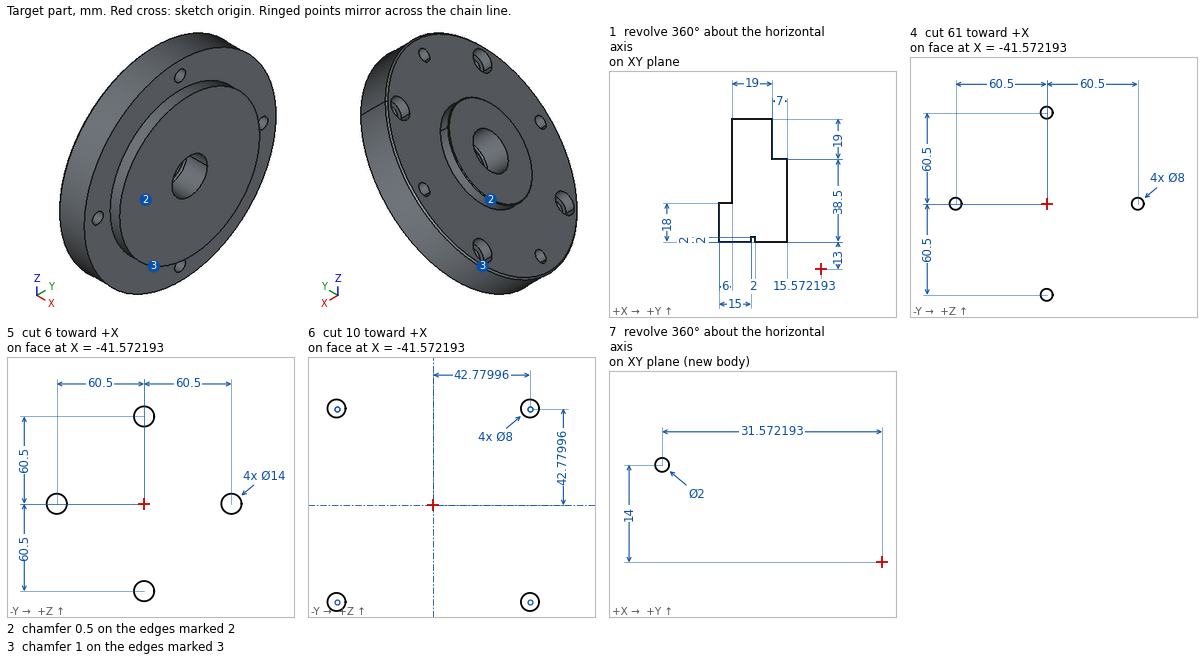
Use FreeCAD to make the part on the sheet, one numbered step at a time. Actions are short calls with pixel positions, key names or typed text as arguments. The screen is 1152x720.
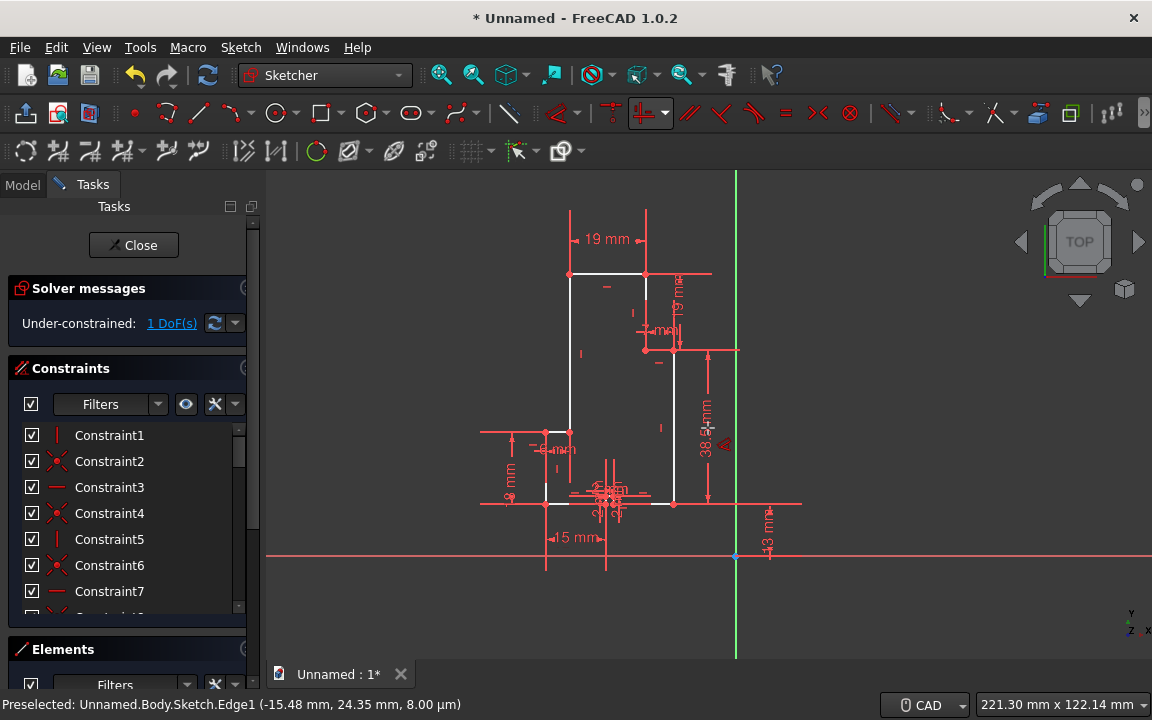
click(674, 504)
click(705, 590)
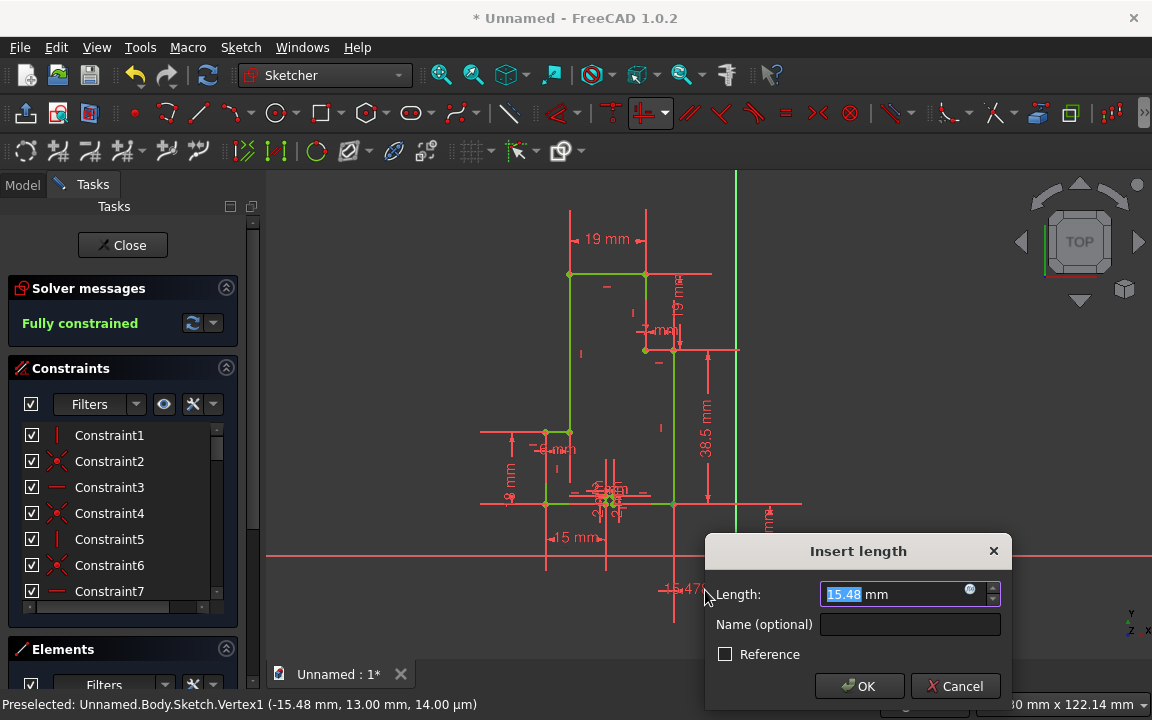
text(15.572193)
key(Return)
key(Escape)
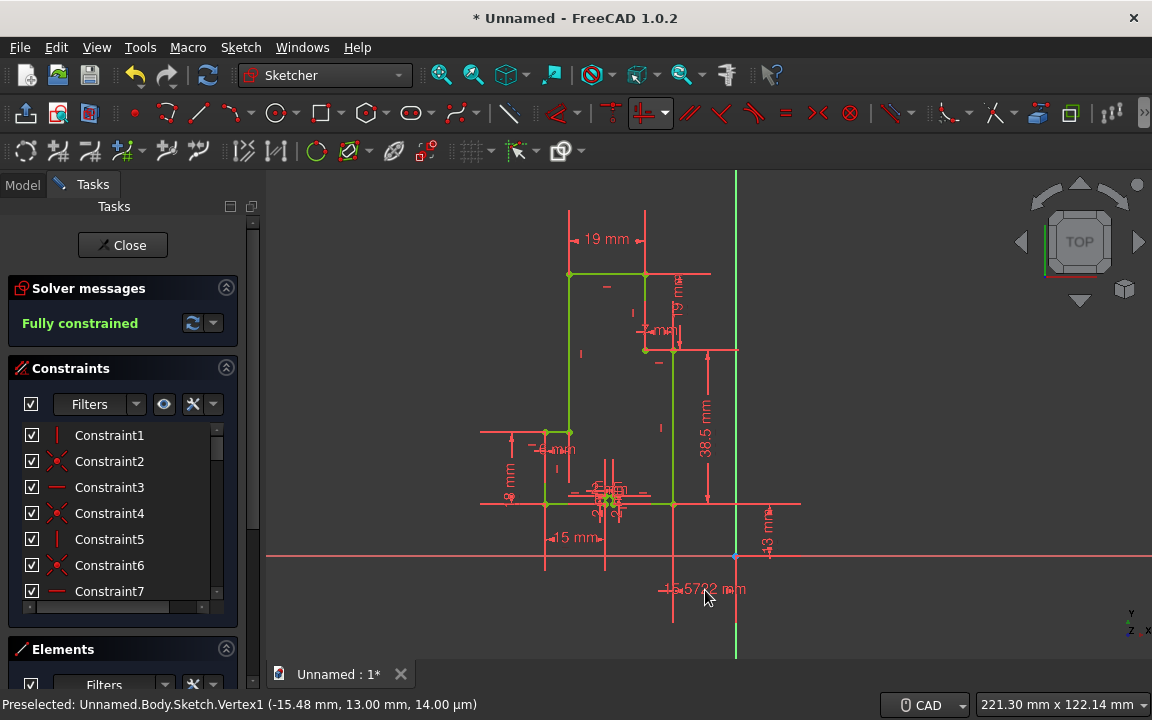
click(123, 245)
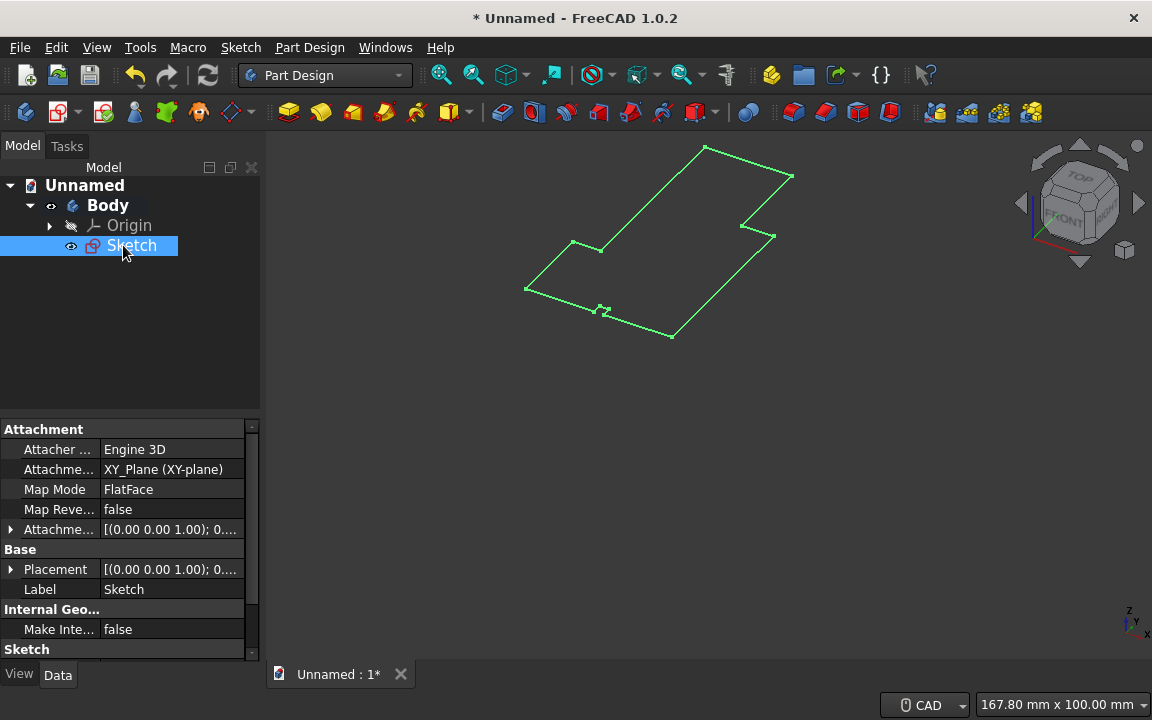
click(322, 112)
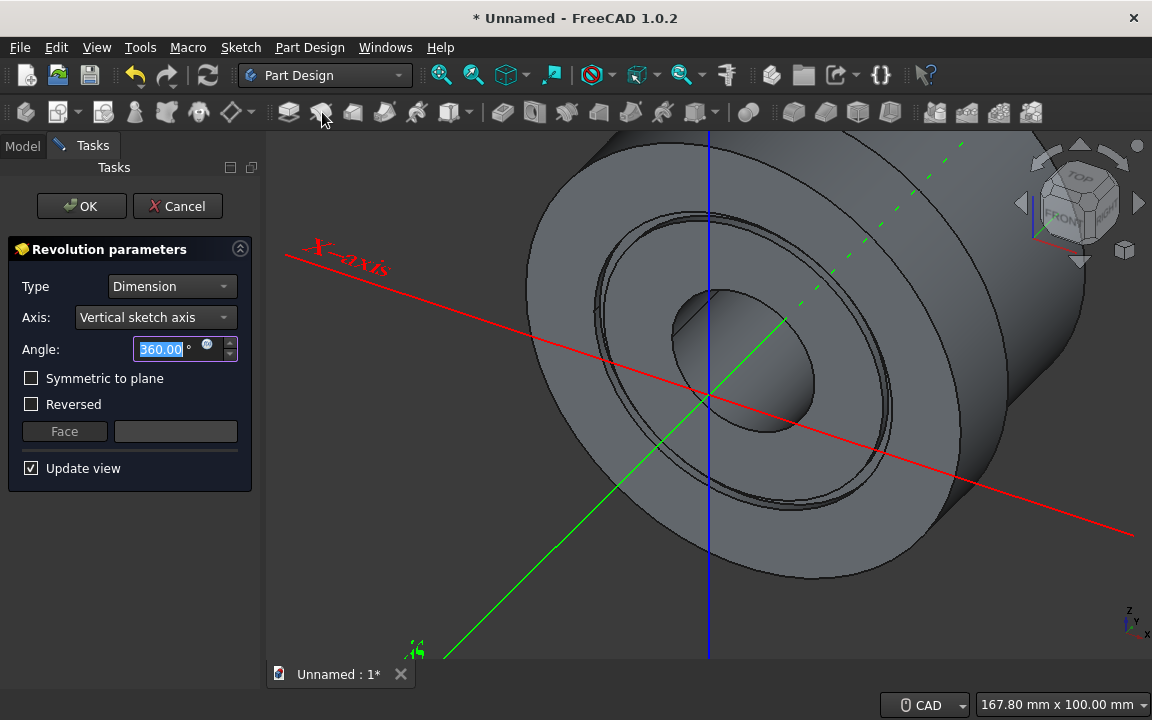
click(156, 318)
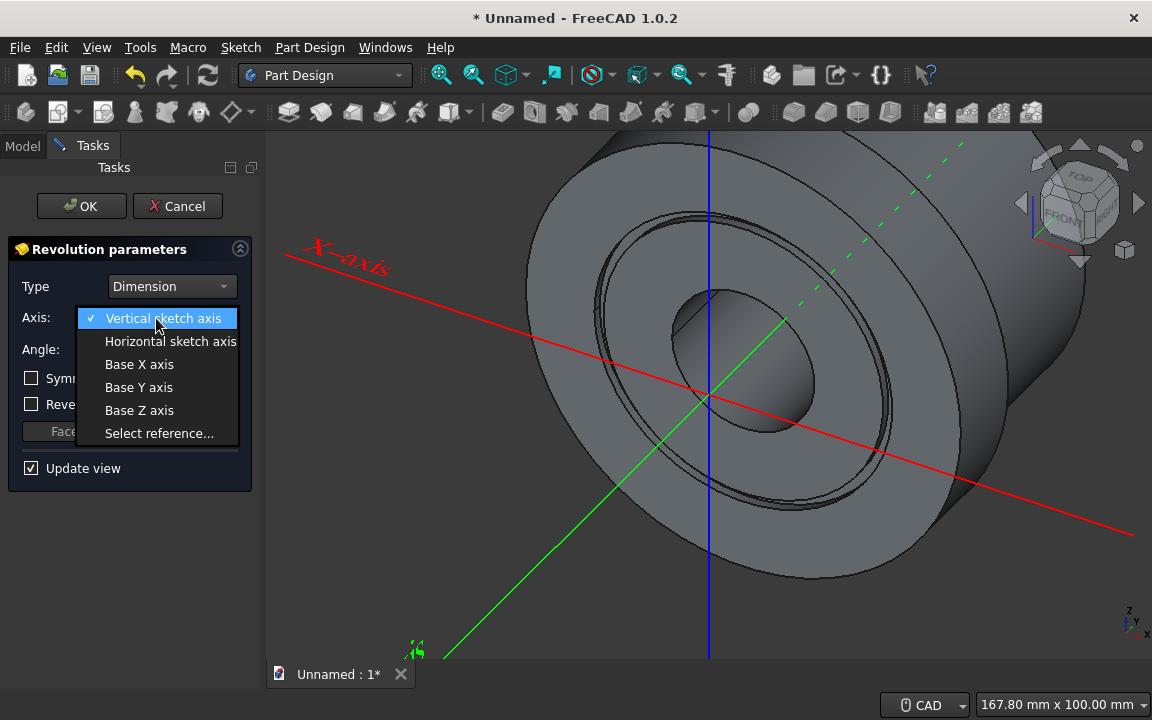
click(156, 342)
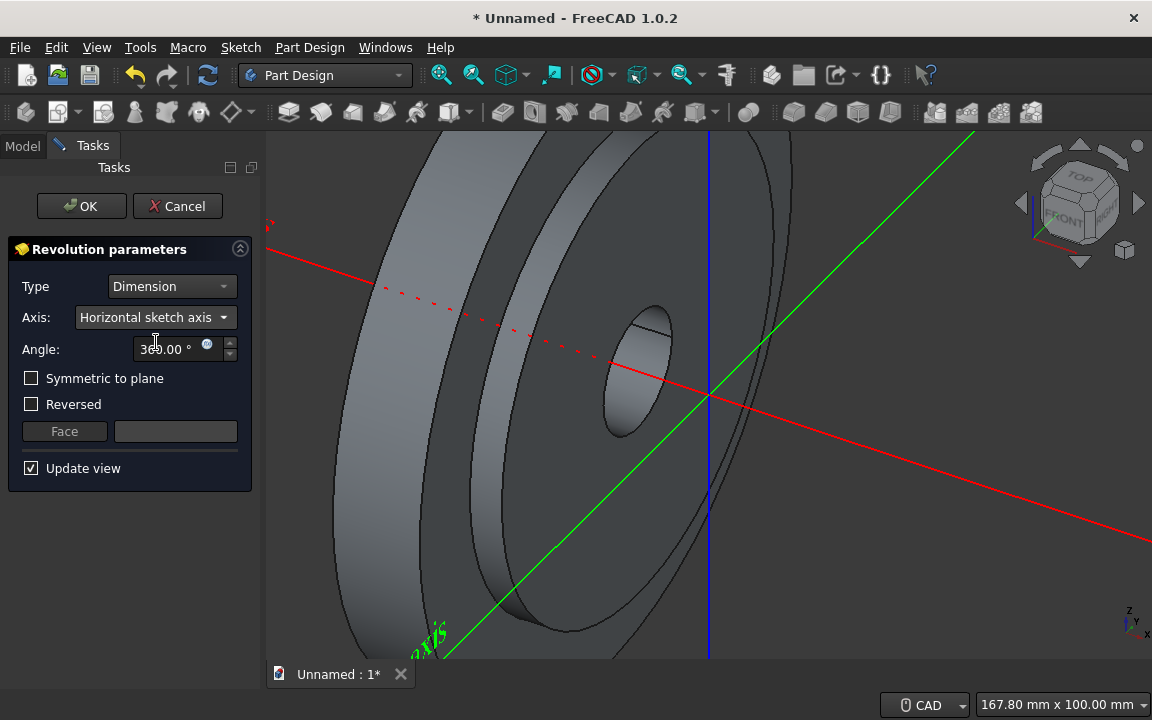
click(82, 206)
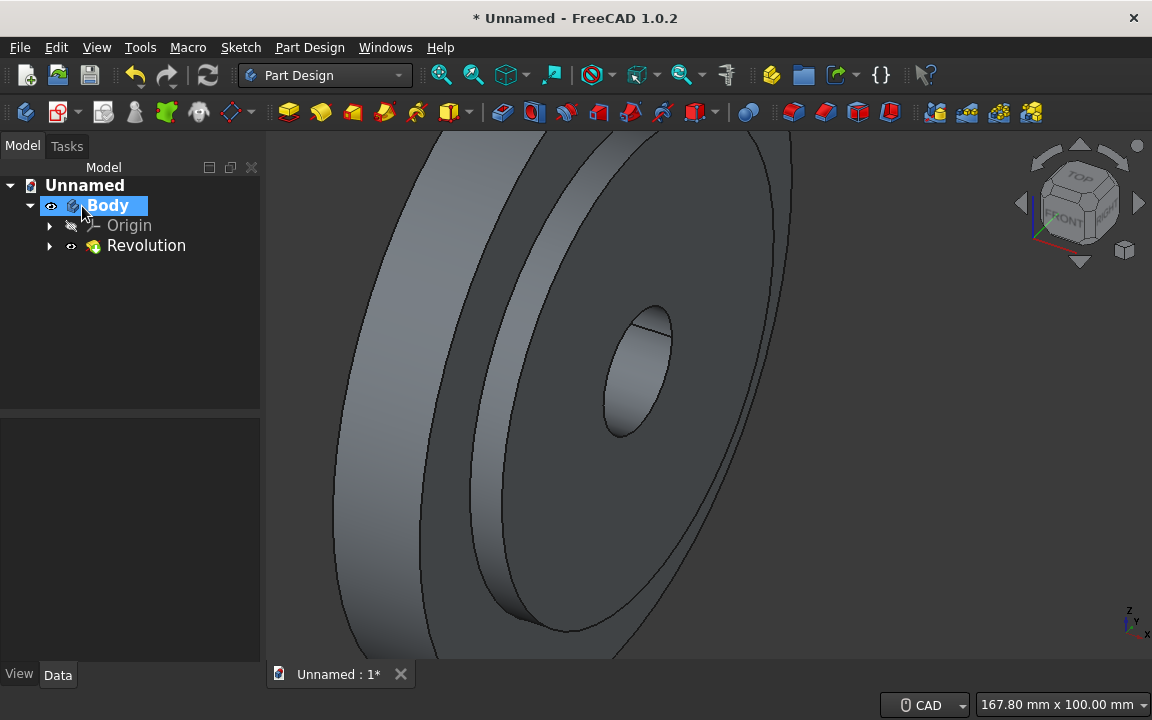
click(442, 76)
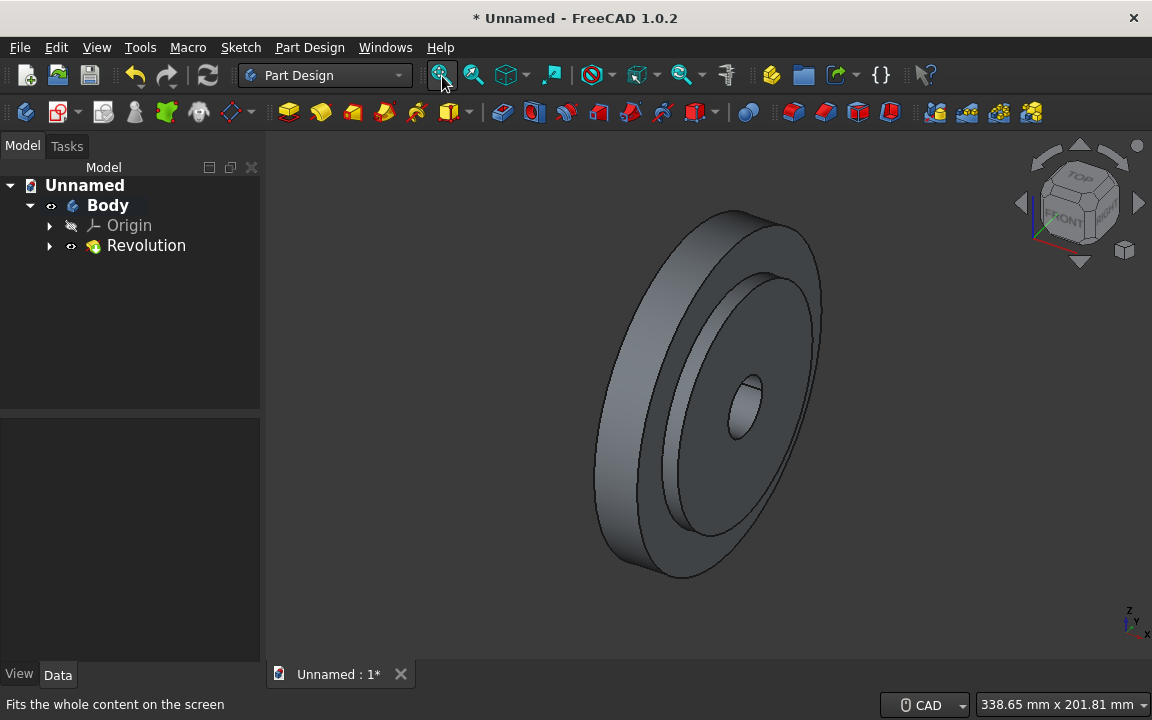
key(0)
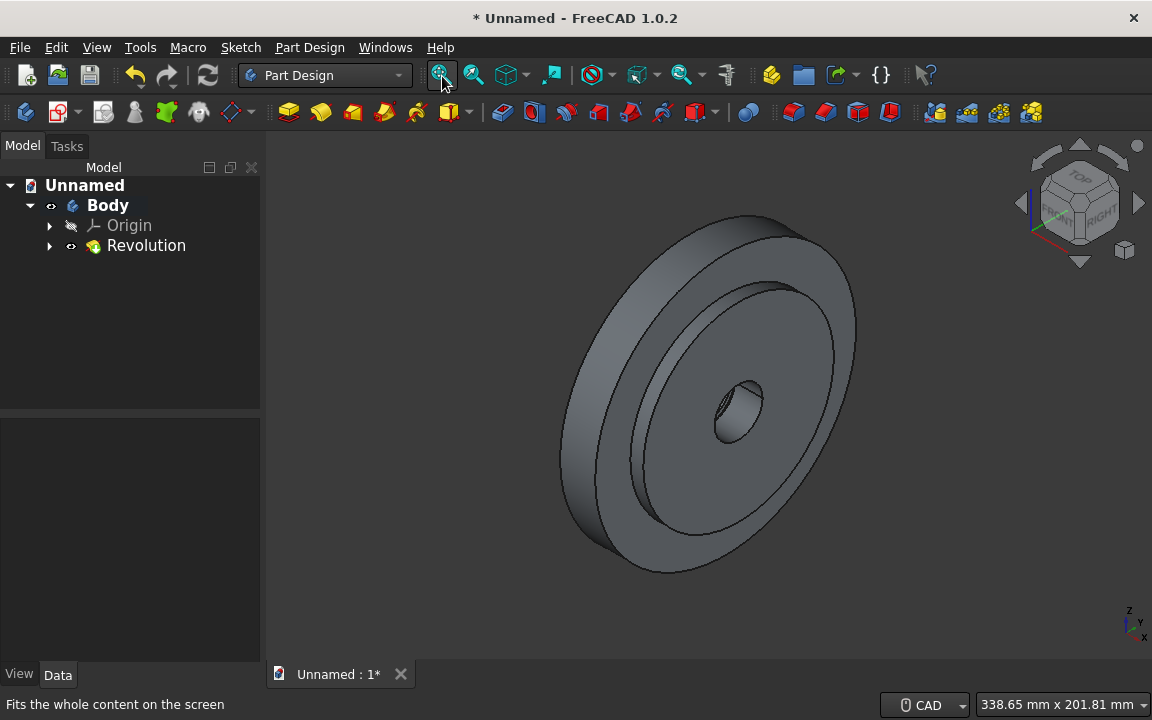
key(2)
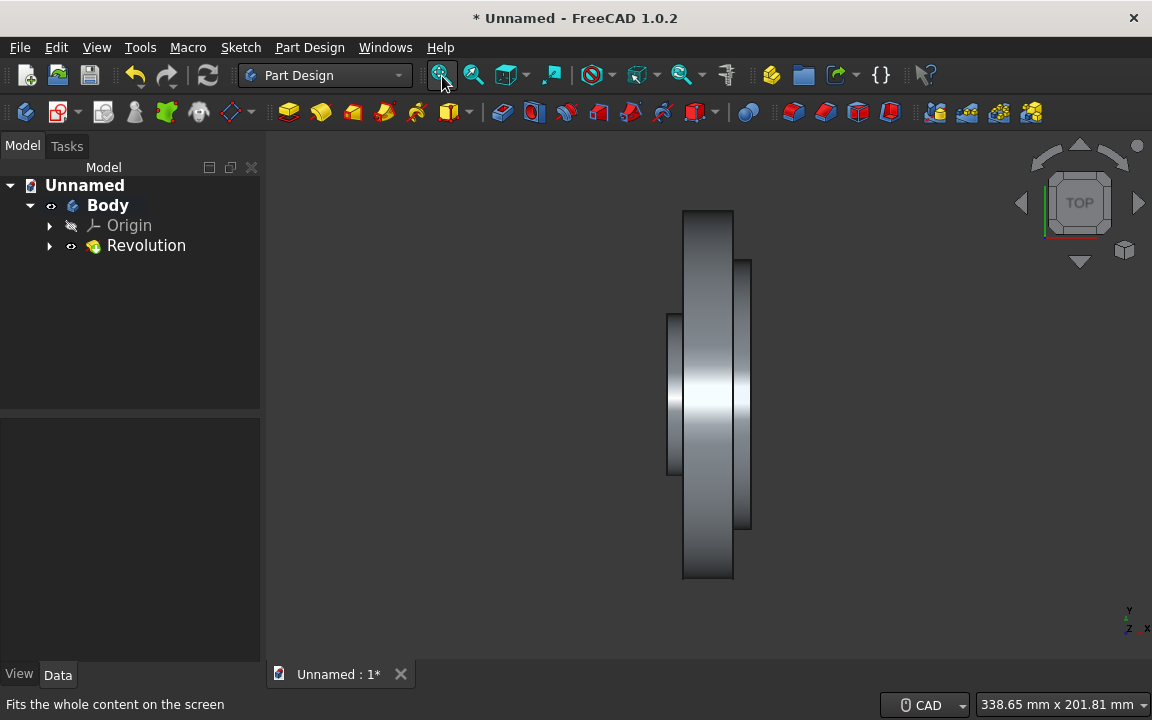
click(667, 460)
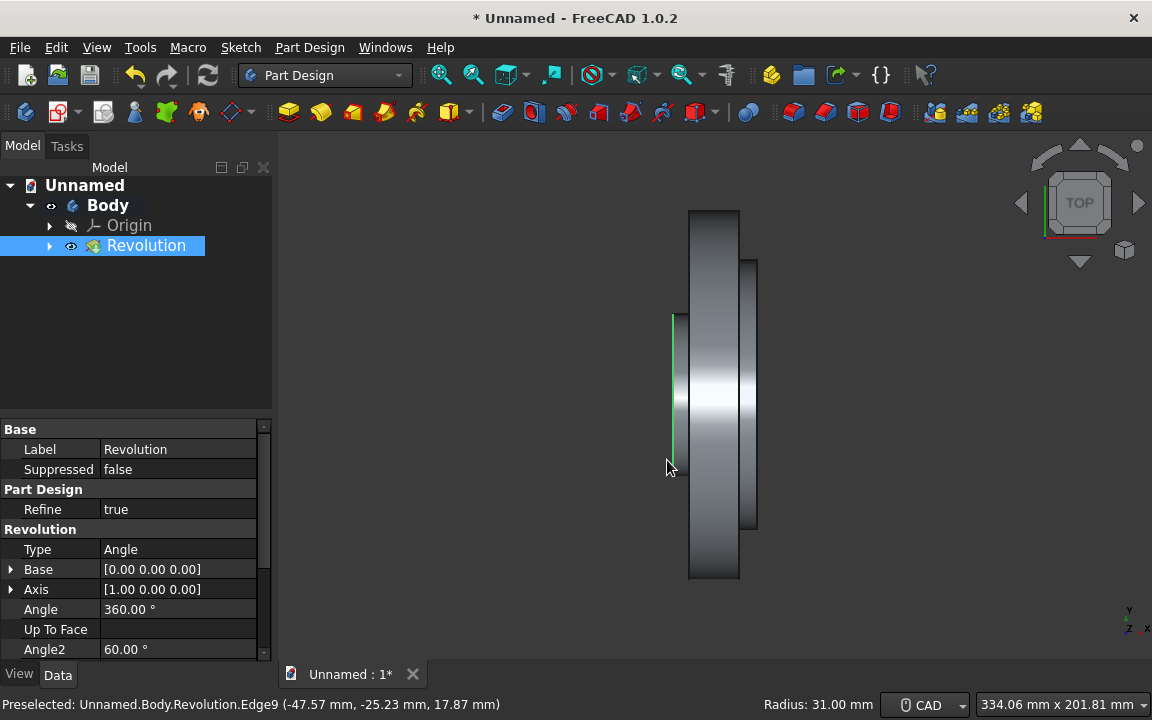
click(826, 112)